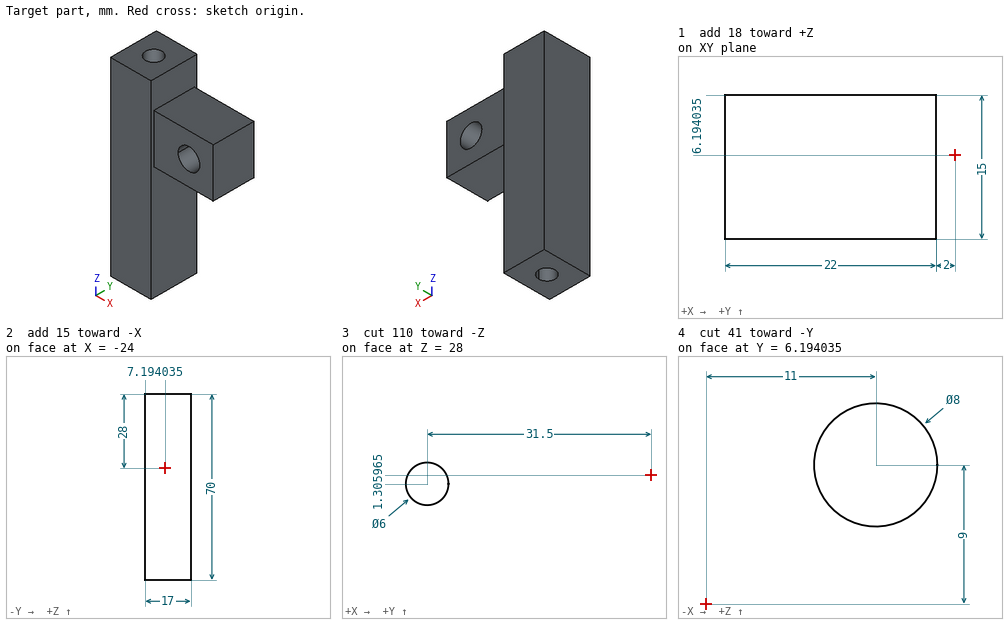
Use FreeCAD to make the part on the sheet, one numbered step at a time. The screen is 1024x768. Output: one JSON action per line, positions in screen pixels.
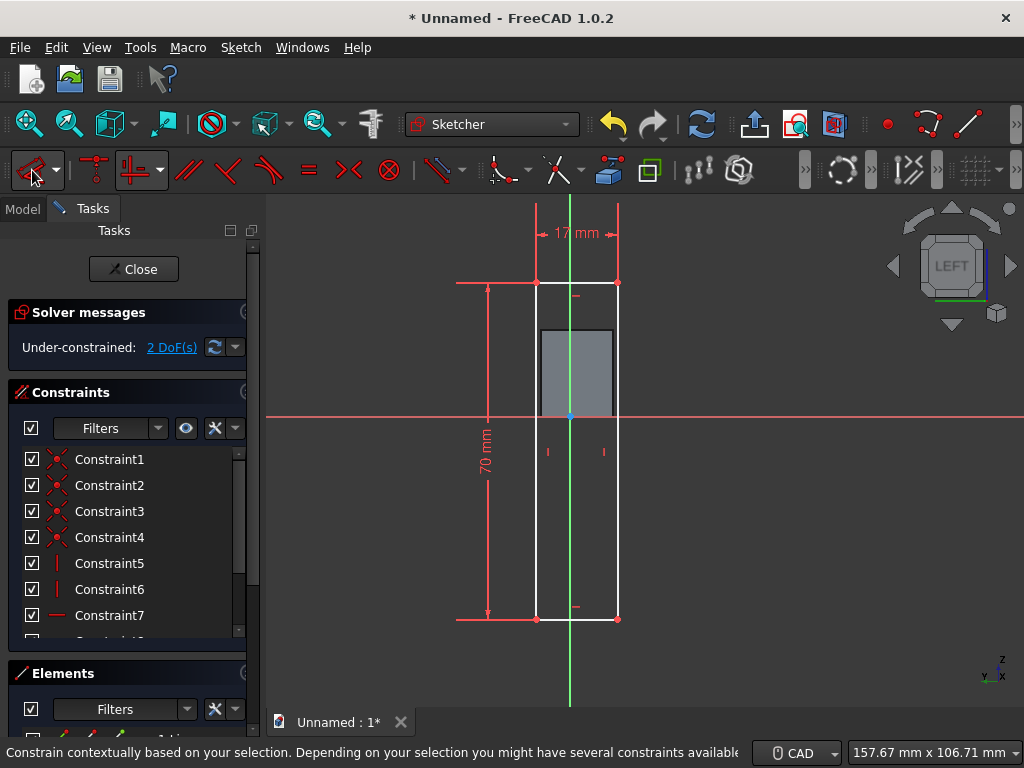
{"action": "left_click", "coordinate": [536, 283]}
{"action": "left_click", "coordinate": [502, 350]}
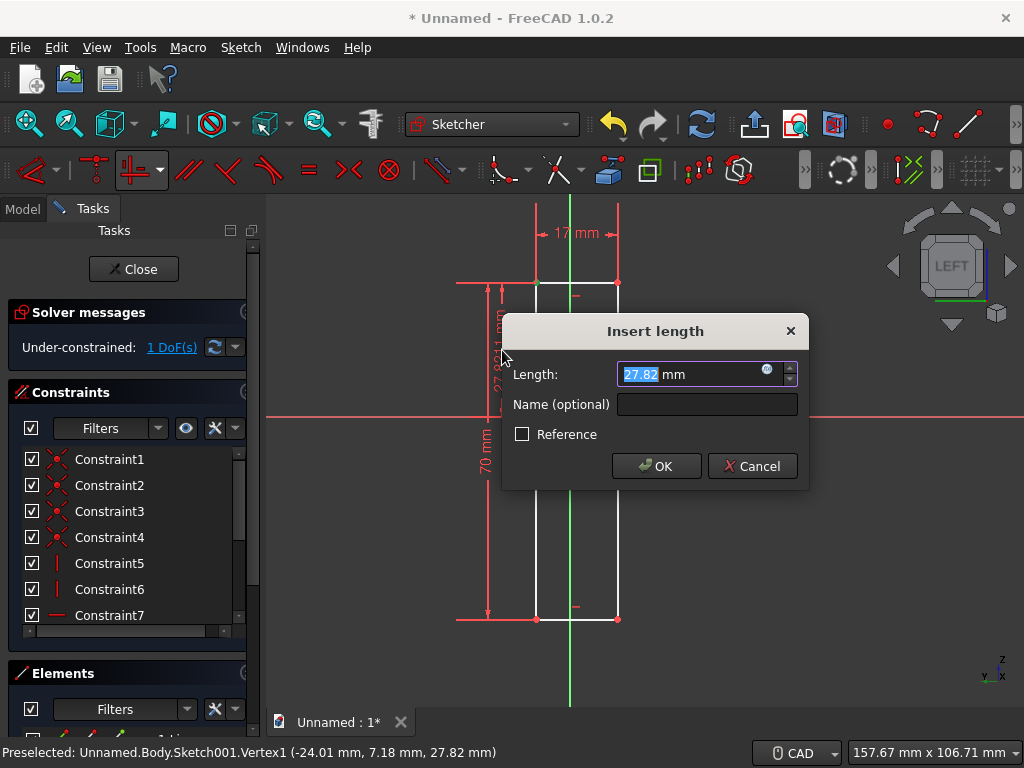
{"action": "type", "text": "28"}
{"action": "key", "text": "Return"}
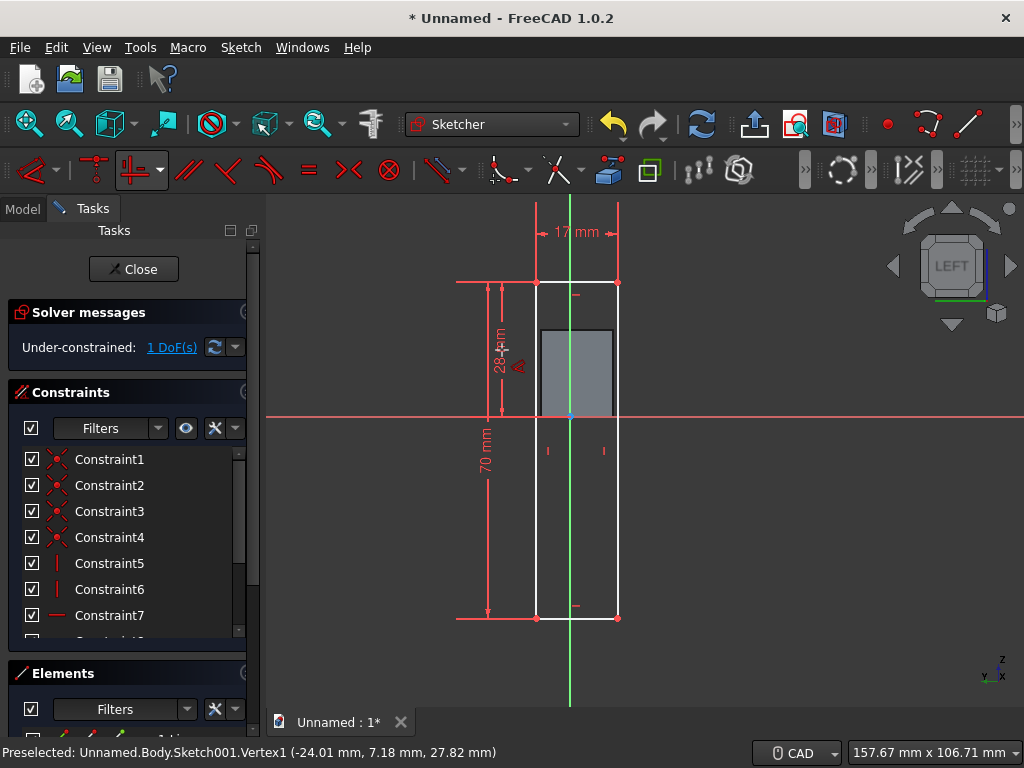
{"action": "left_click", "coordinate": [536, 282]}
{"action": "left_click", "coordinate": [553, 248]}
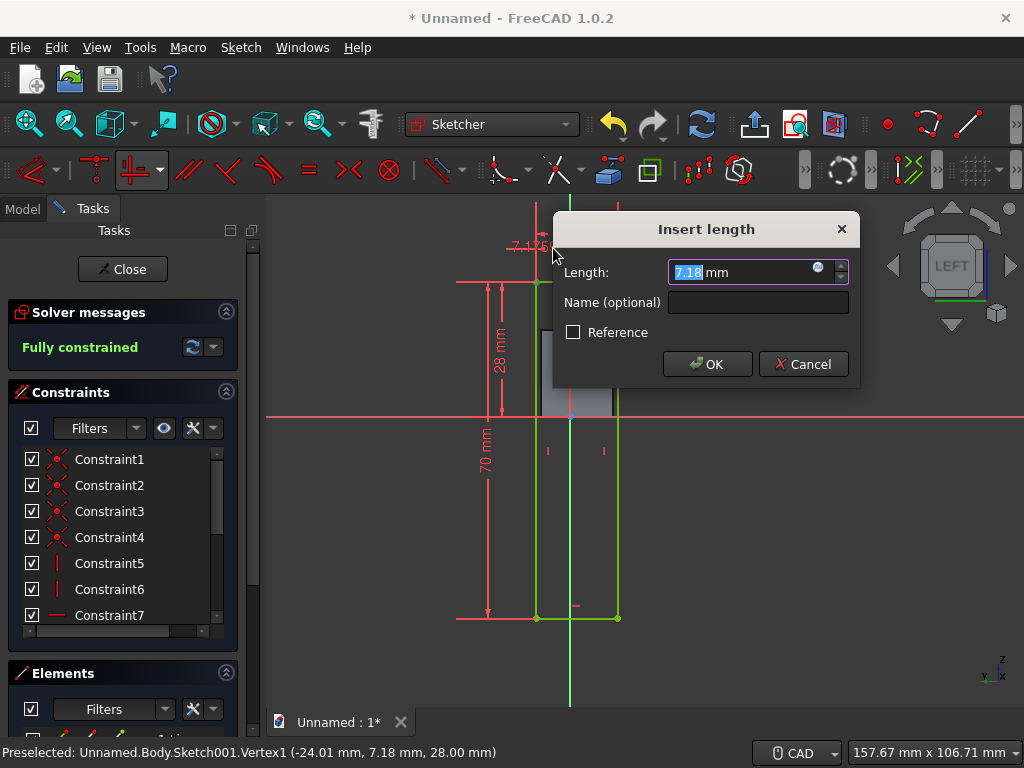
{"action": "type", "text": "7.194035"}
{"action": "key", "text": "Return"}
{"action": "key", "text": "Escape"}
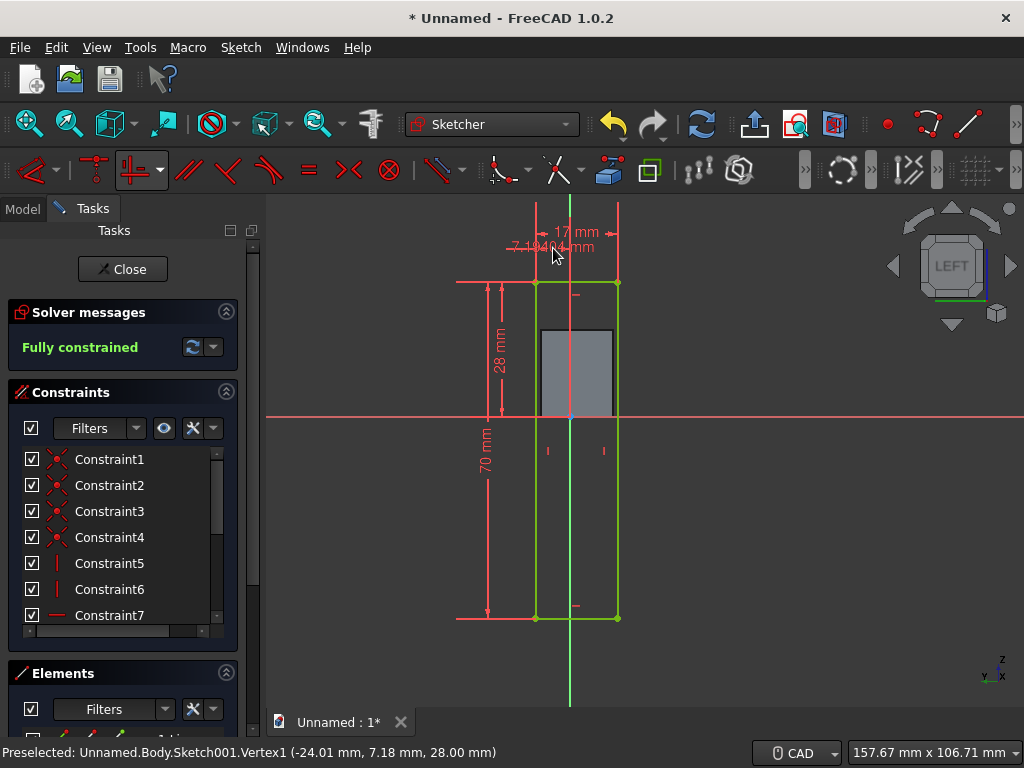
{"action": "left_click", "coordinate": [123, 269]}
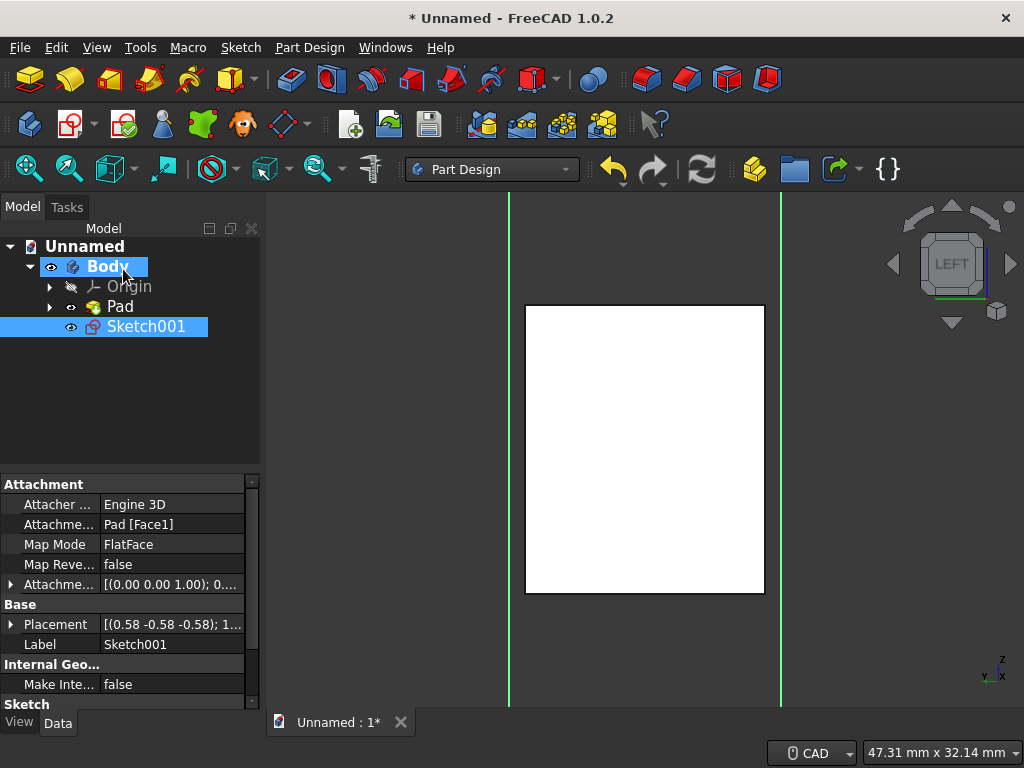
{"action": "left_click", "coordinate": [30, 80]}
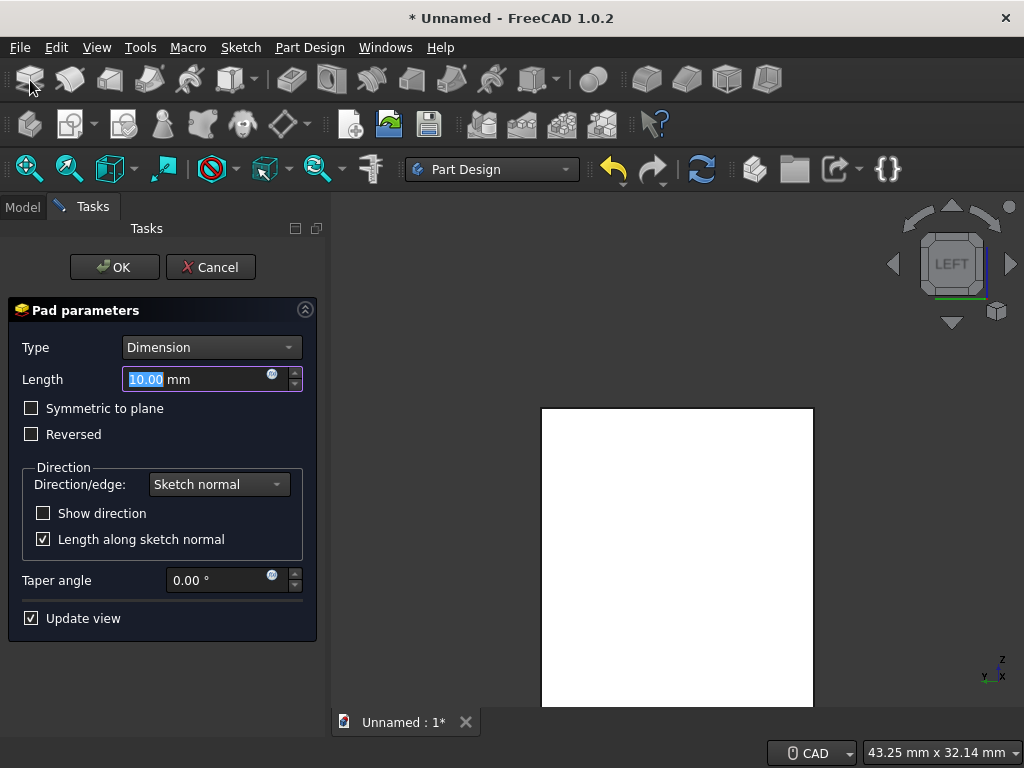
{"action": "type", "text": "15"}
{"action": "key", "text": "Tab"}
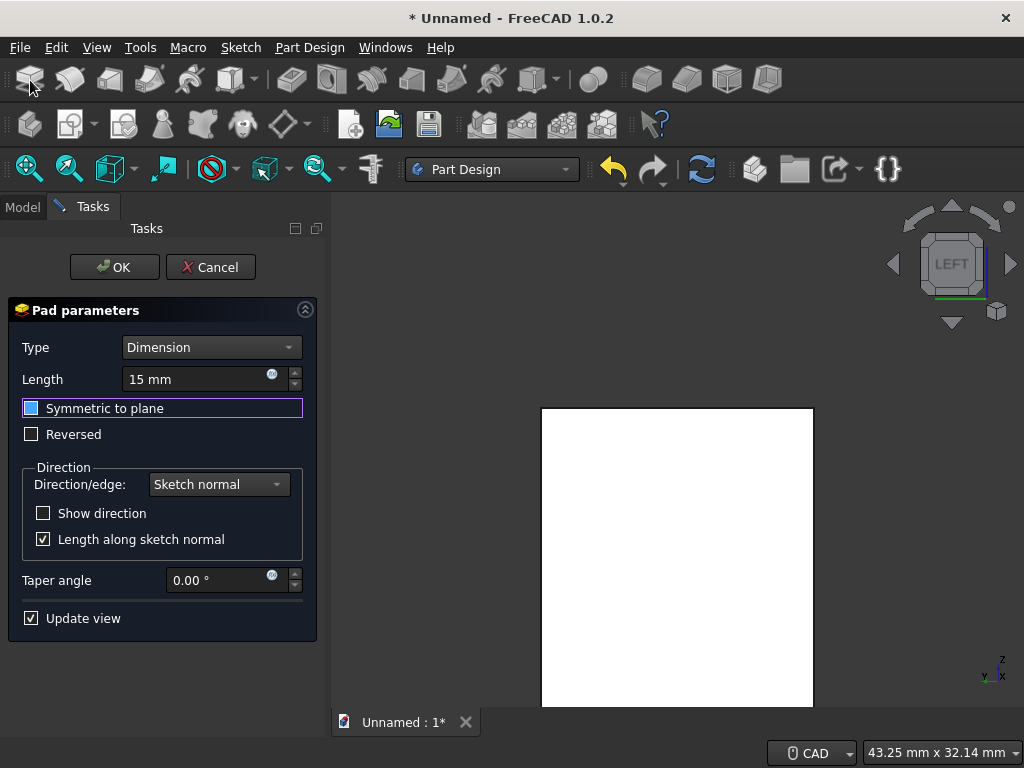
{"action": "left_click", "coordinate": [115, 267]}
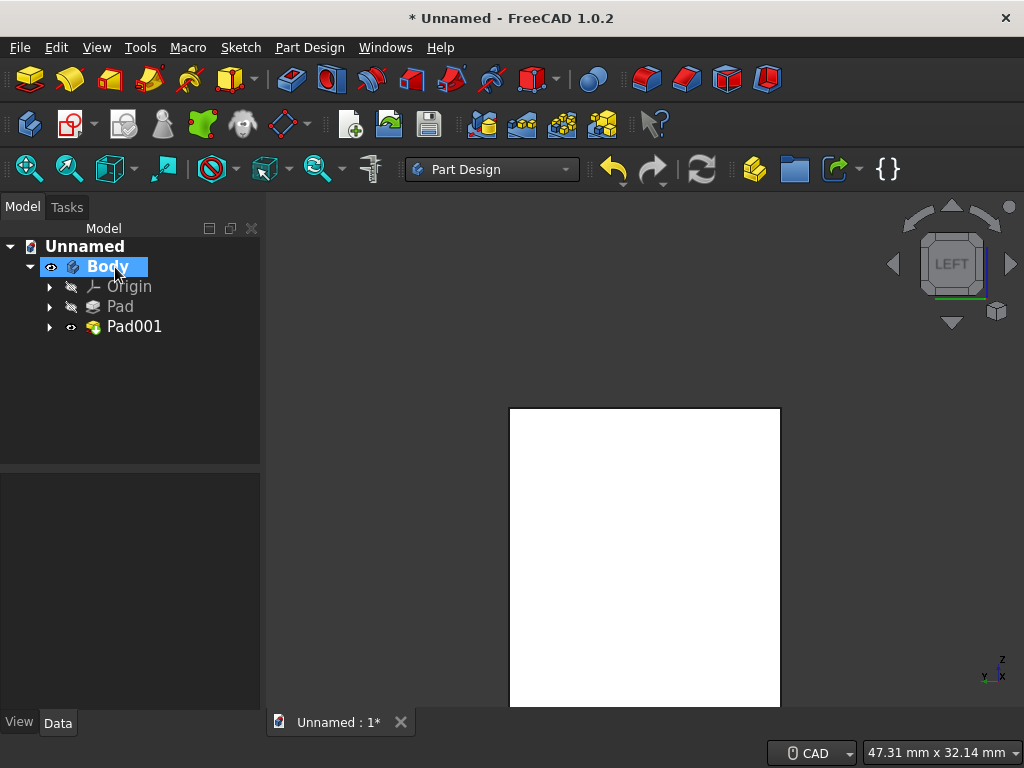
{"action": "left_click", "coordinate": [30, 170]}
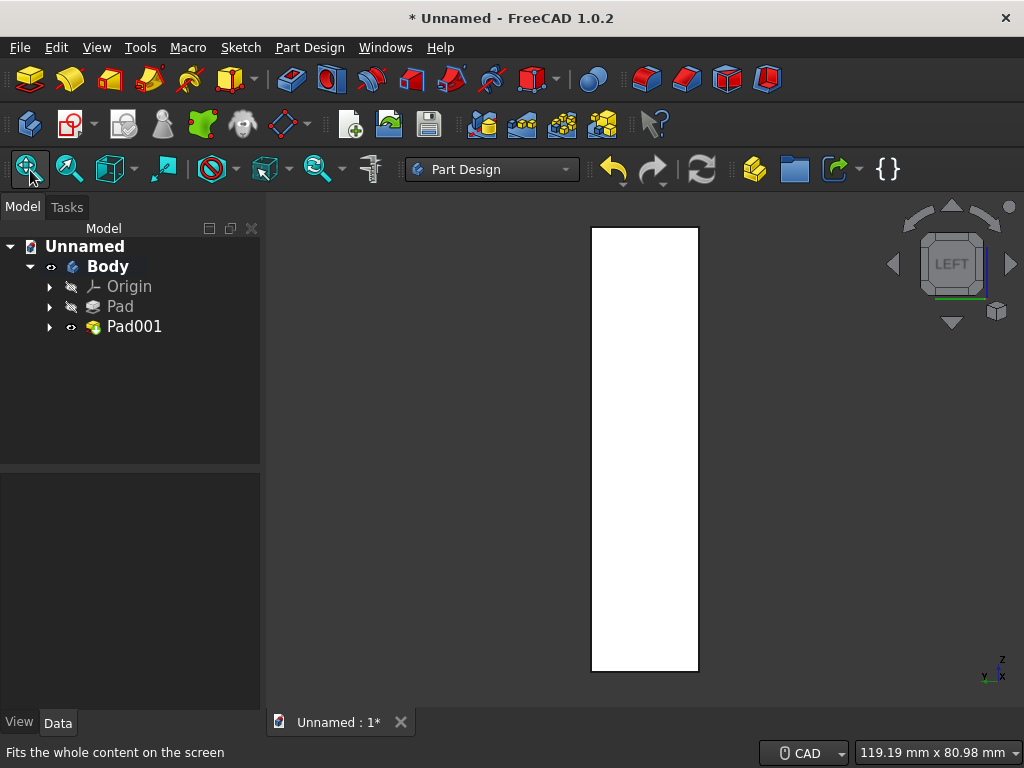
{"action": "key", "text": "0"}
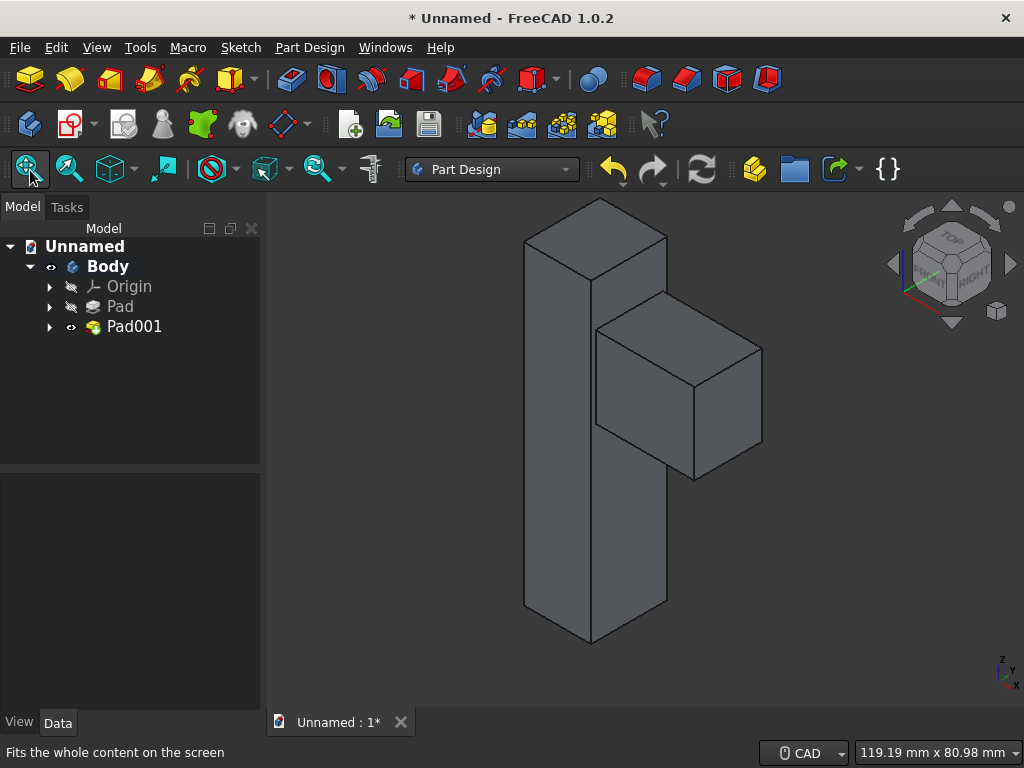
{"action": "left_click", "coordinate": [596, 238]}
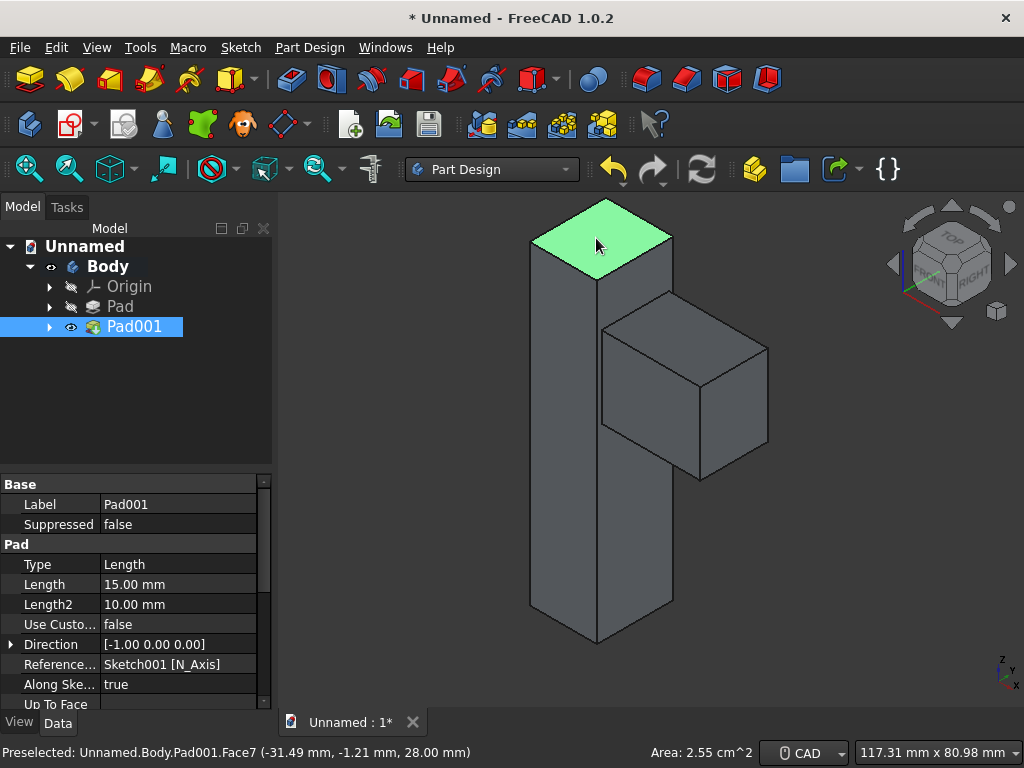
{"action": "left_click", "coordinate": [70, 124]}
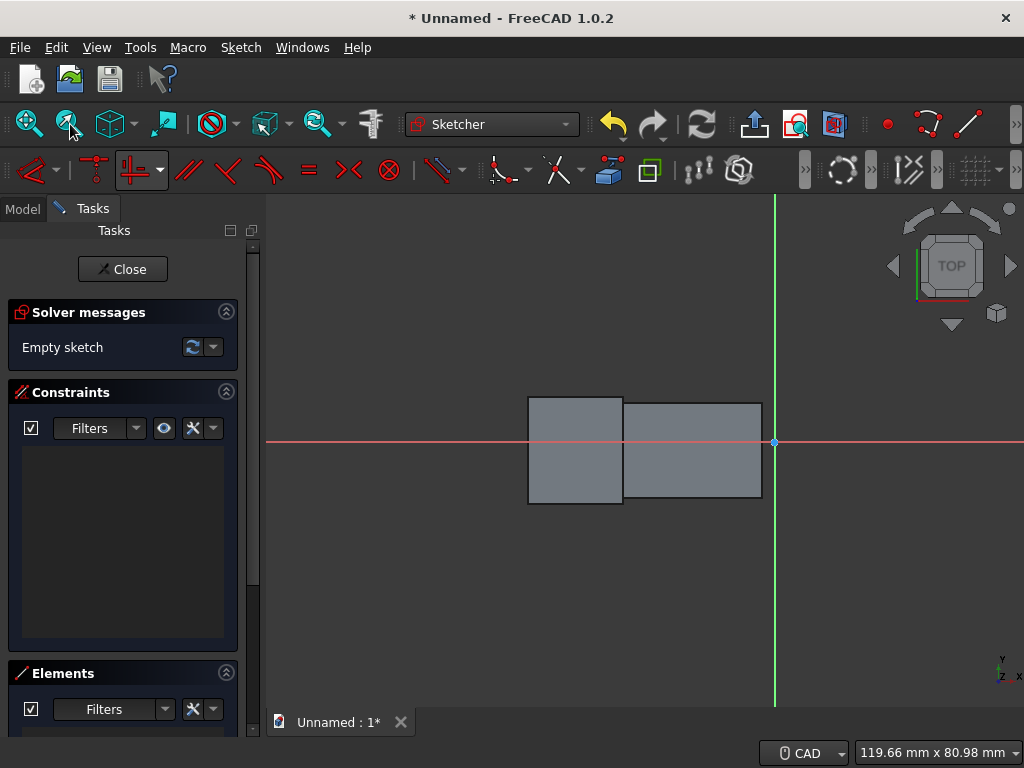
{"action": "scroll", "coordinate": [575, 451], "scroll_direction": "up", "scroll_amount": 11}